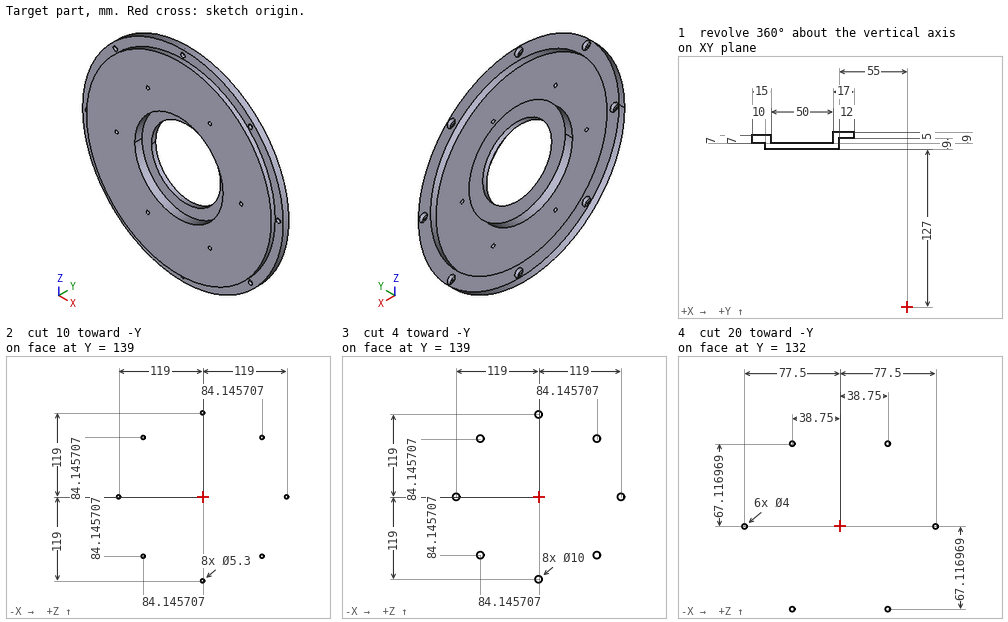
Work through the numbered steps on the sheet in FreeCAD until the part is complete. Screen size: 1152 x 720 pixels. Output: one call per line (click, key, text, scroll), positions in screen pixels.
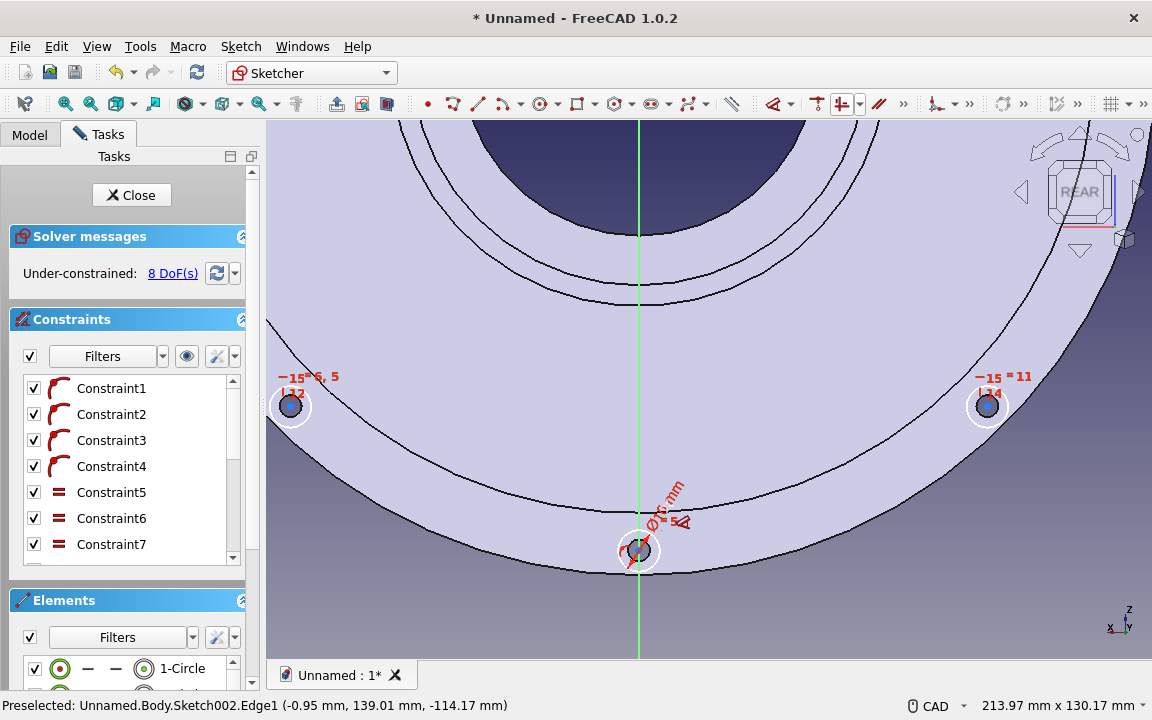
click(639, 551)
click(673, 349)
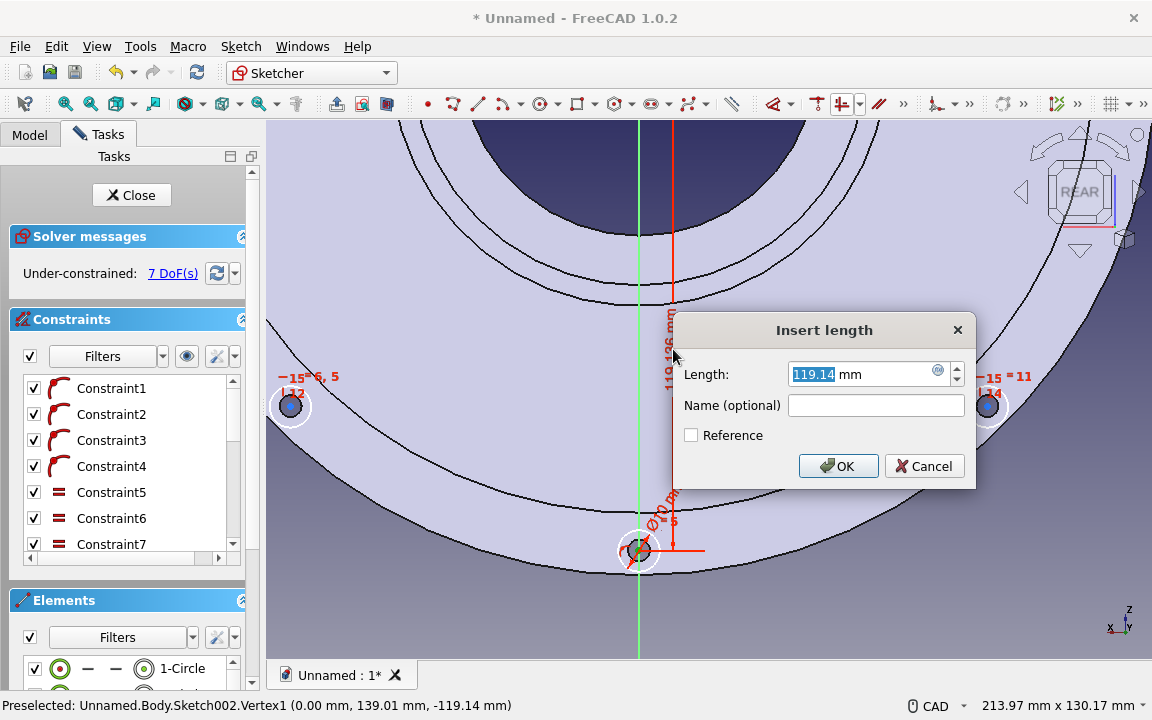
text(119)
key(Return)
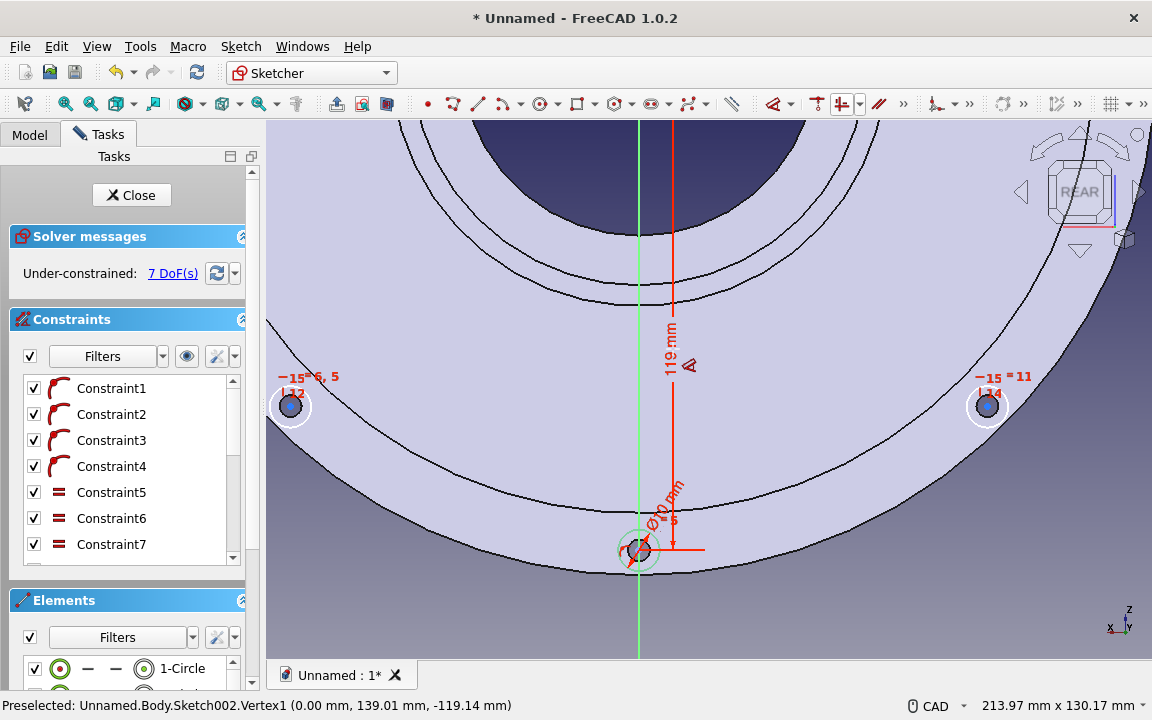
scroll(641, 533, down, 6)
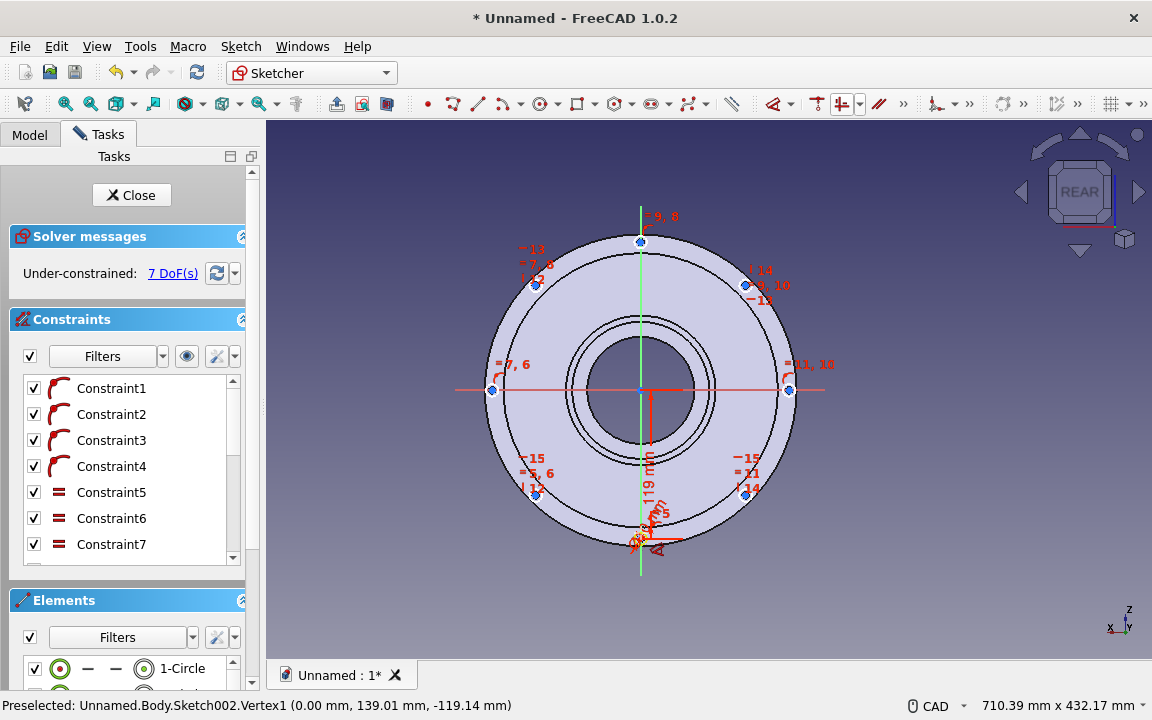
click(492, 390)
click(566, 424)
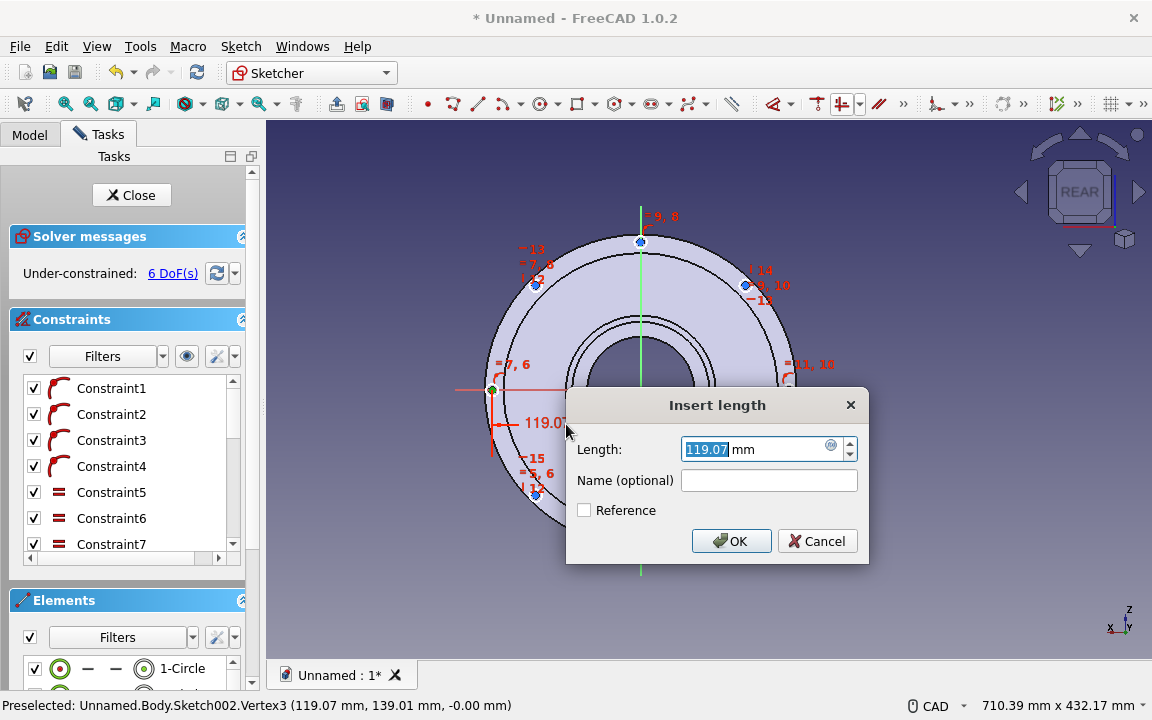
text(119)
key(Return)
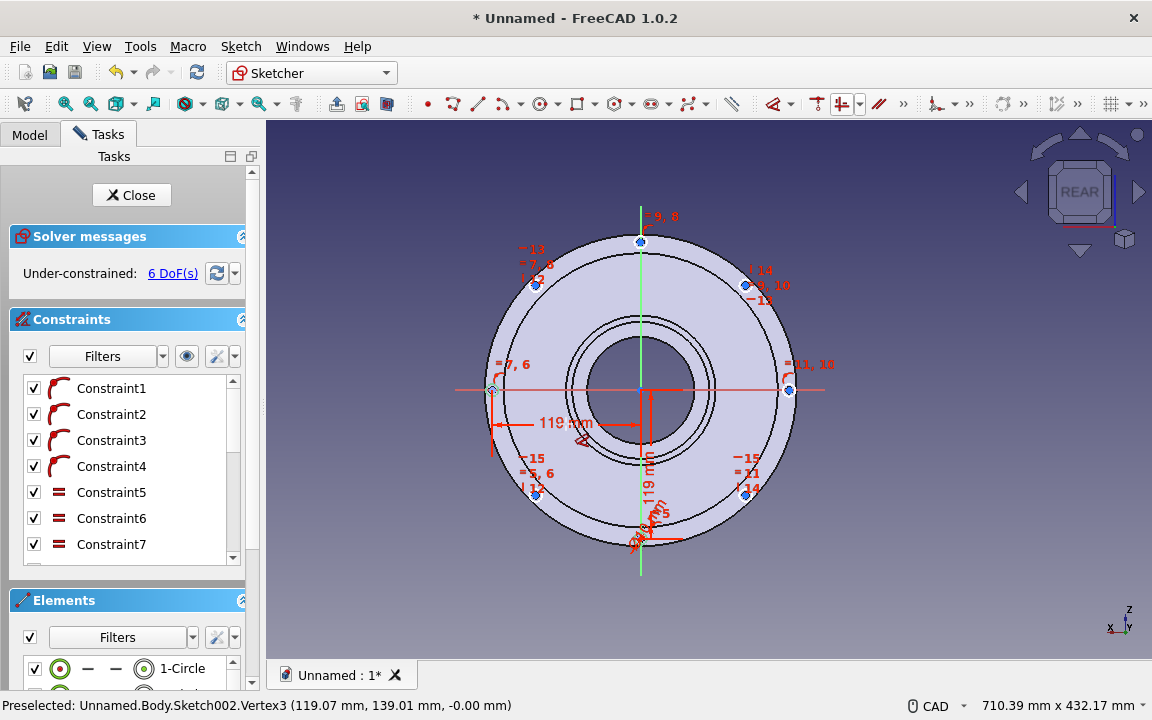
click(641, 242)
click(675, 316)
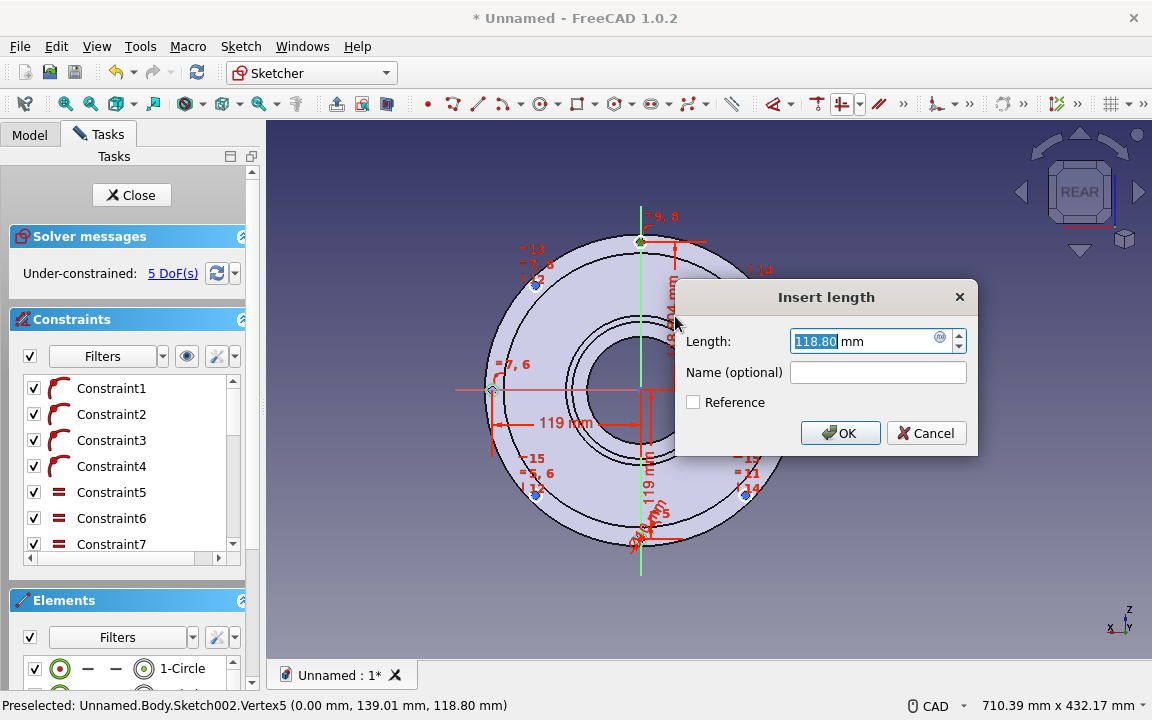
text(119)
key(Return)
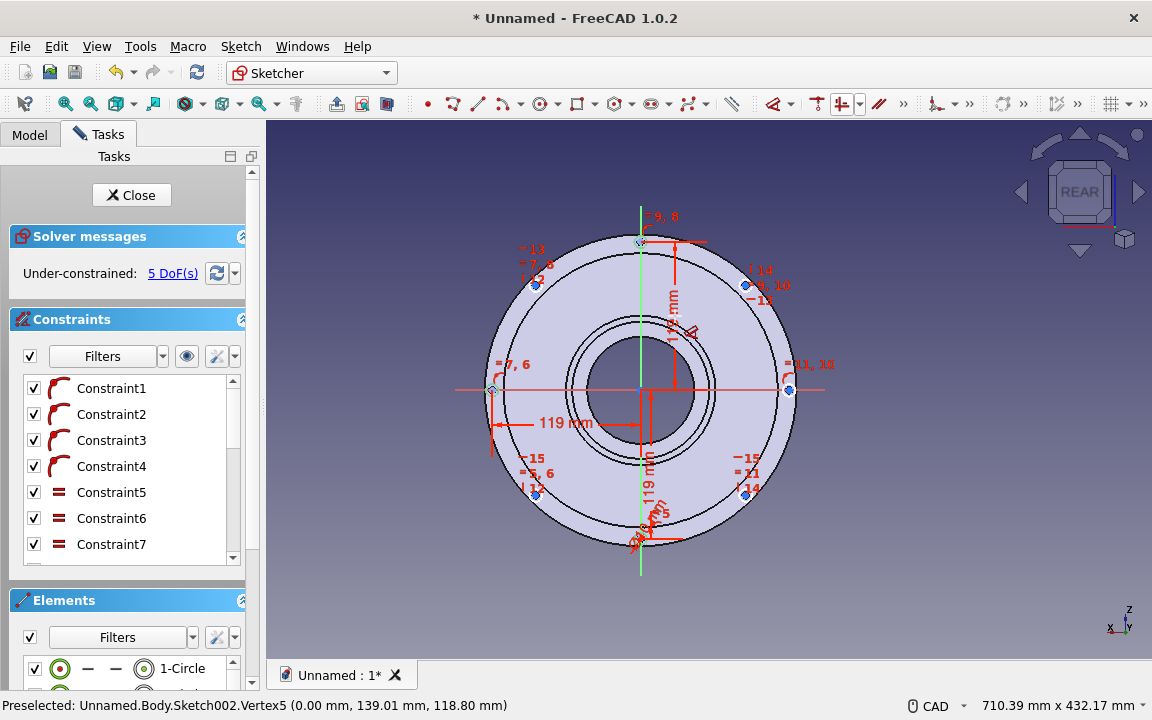
click(789, 390)
click(715, 424)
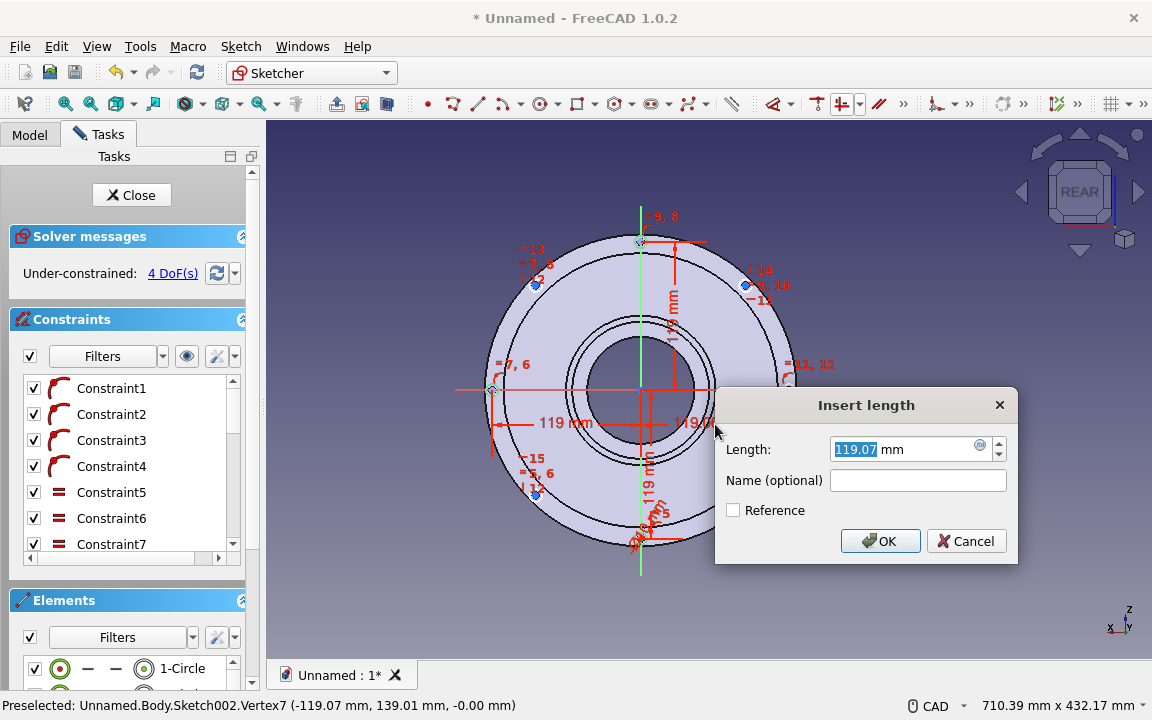
text(119)
key(Return)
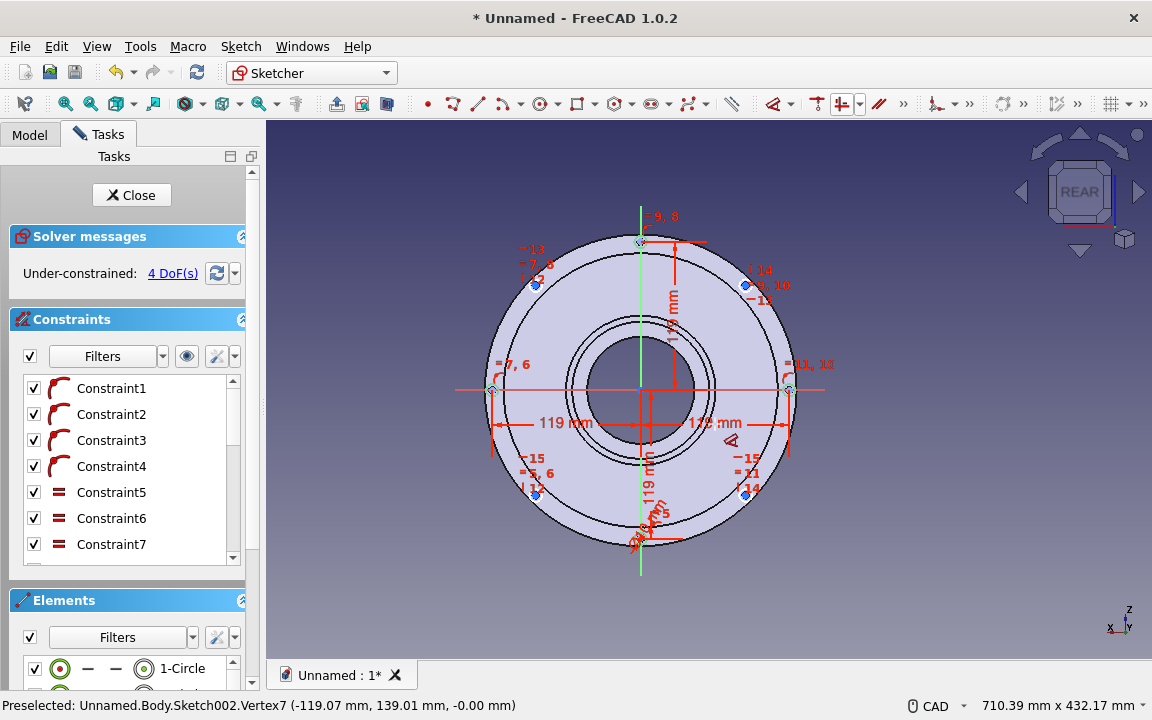
click(536, 496)
click(564, 530)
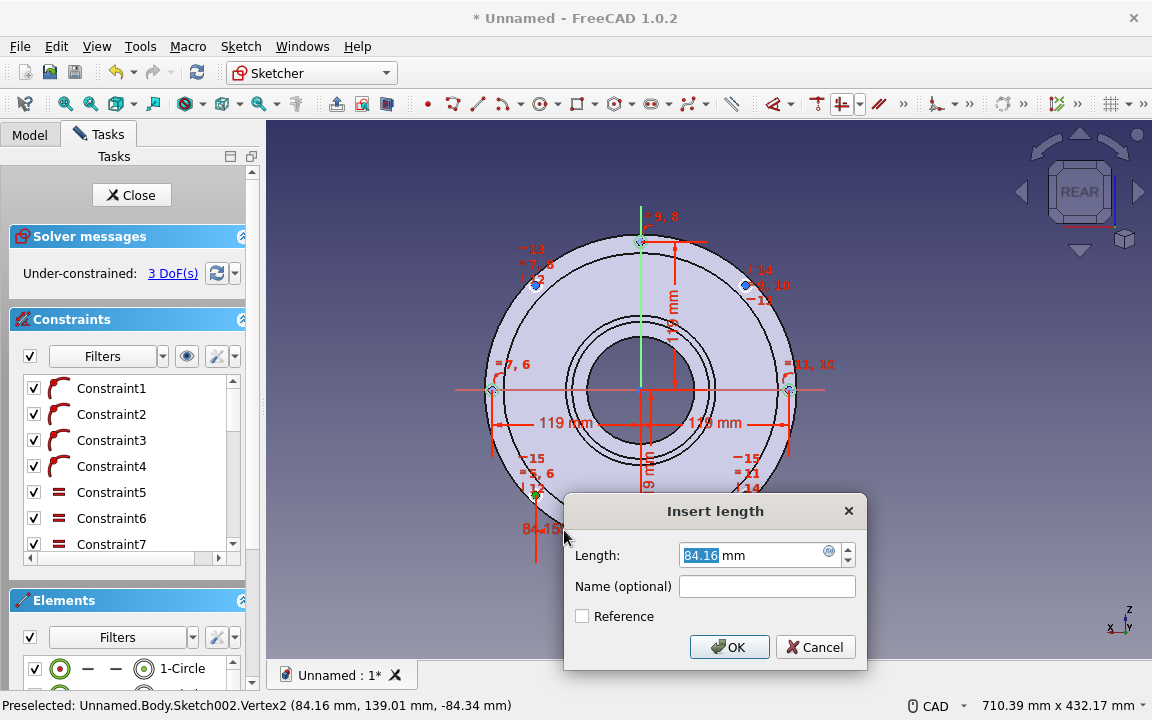
text(84.145707)
key(Return)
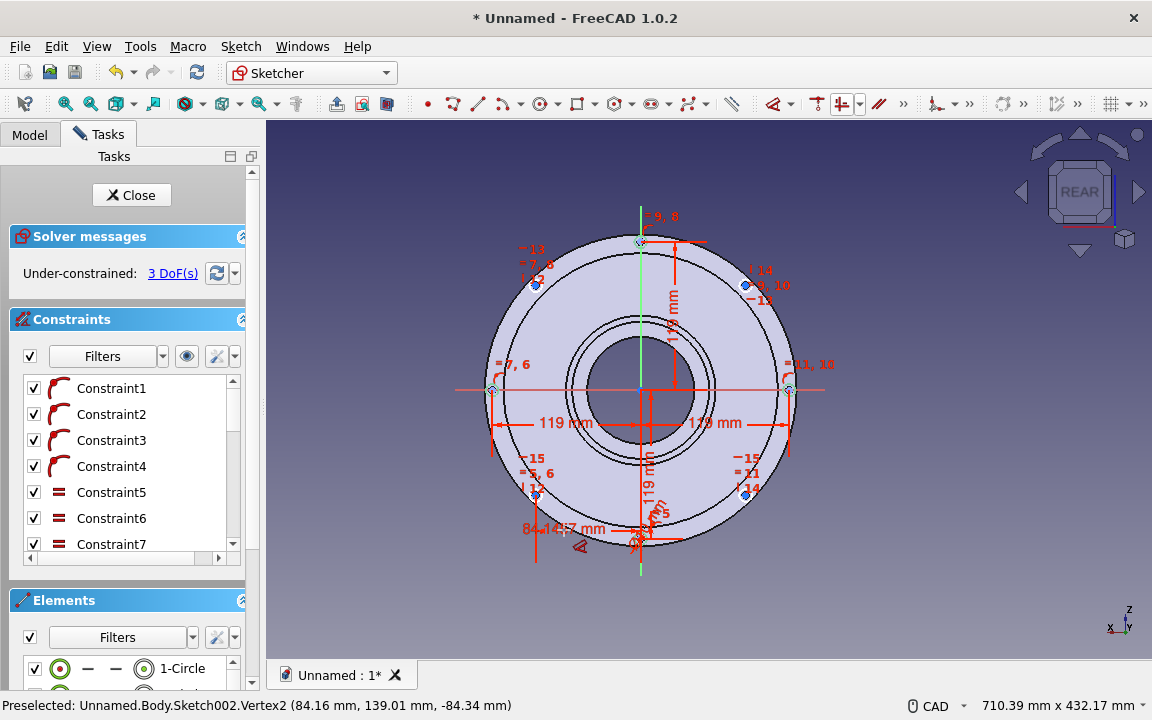
click(536, 496)
click(502, 467)